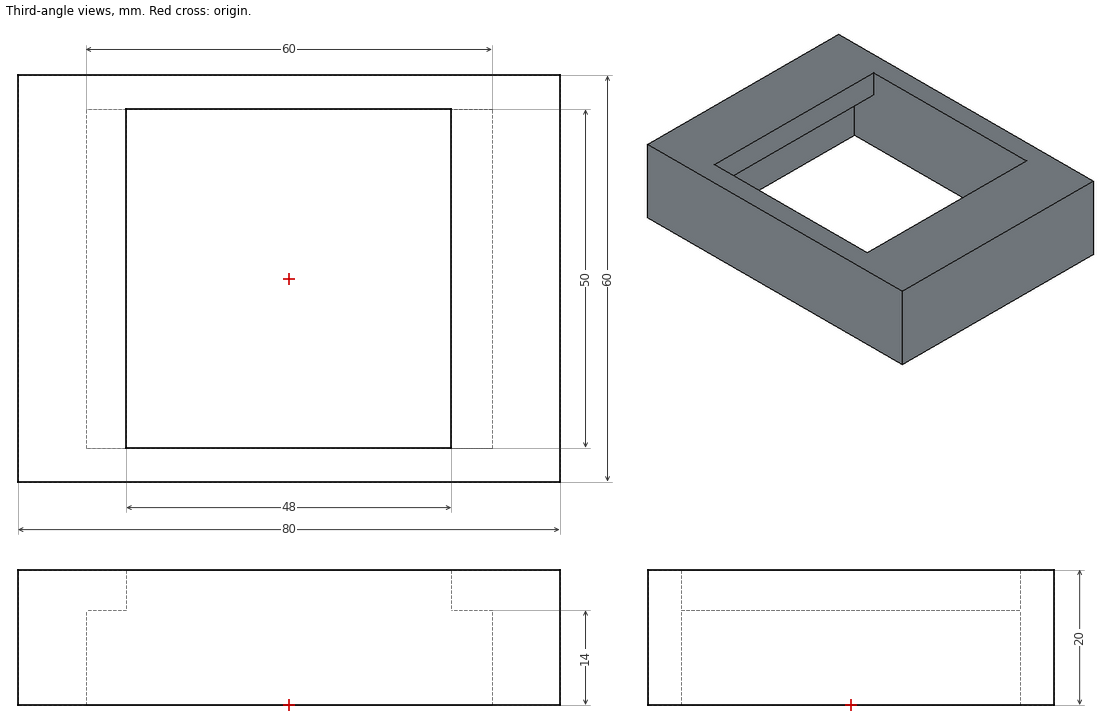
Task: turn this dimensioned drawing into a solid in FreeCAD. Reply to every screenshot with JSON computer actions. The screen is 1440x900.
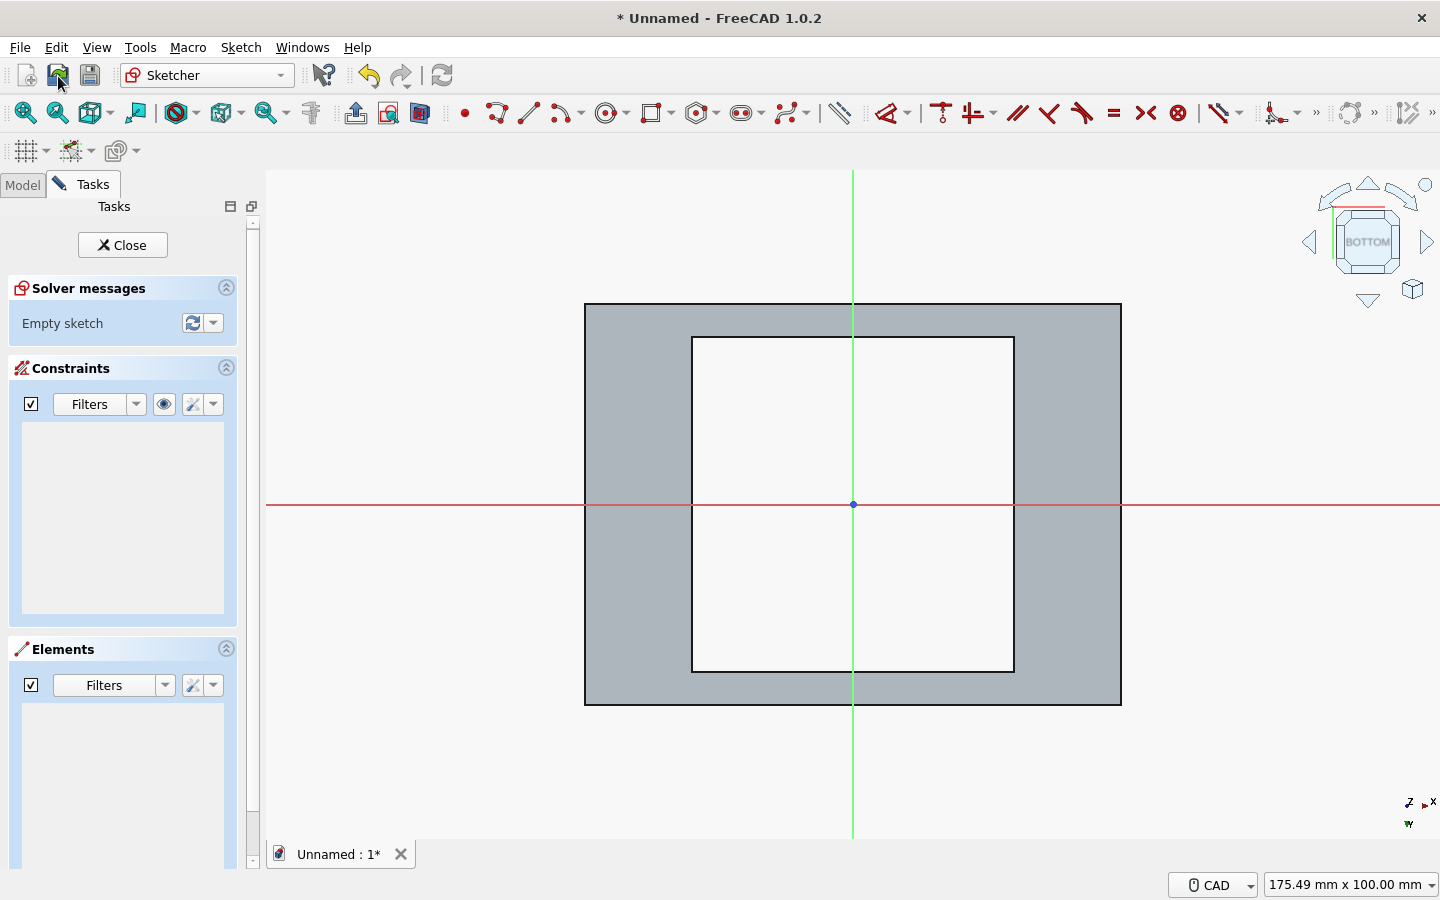
{"action": "key", "text": "g v"}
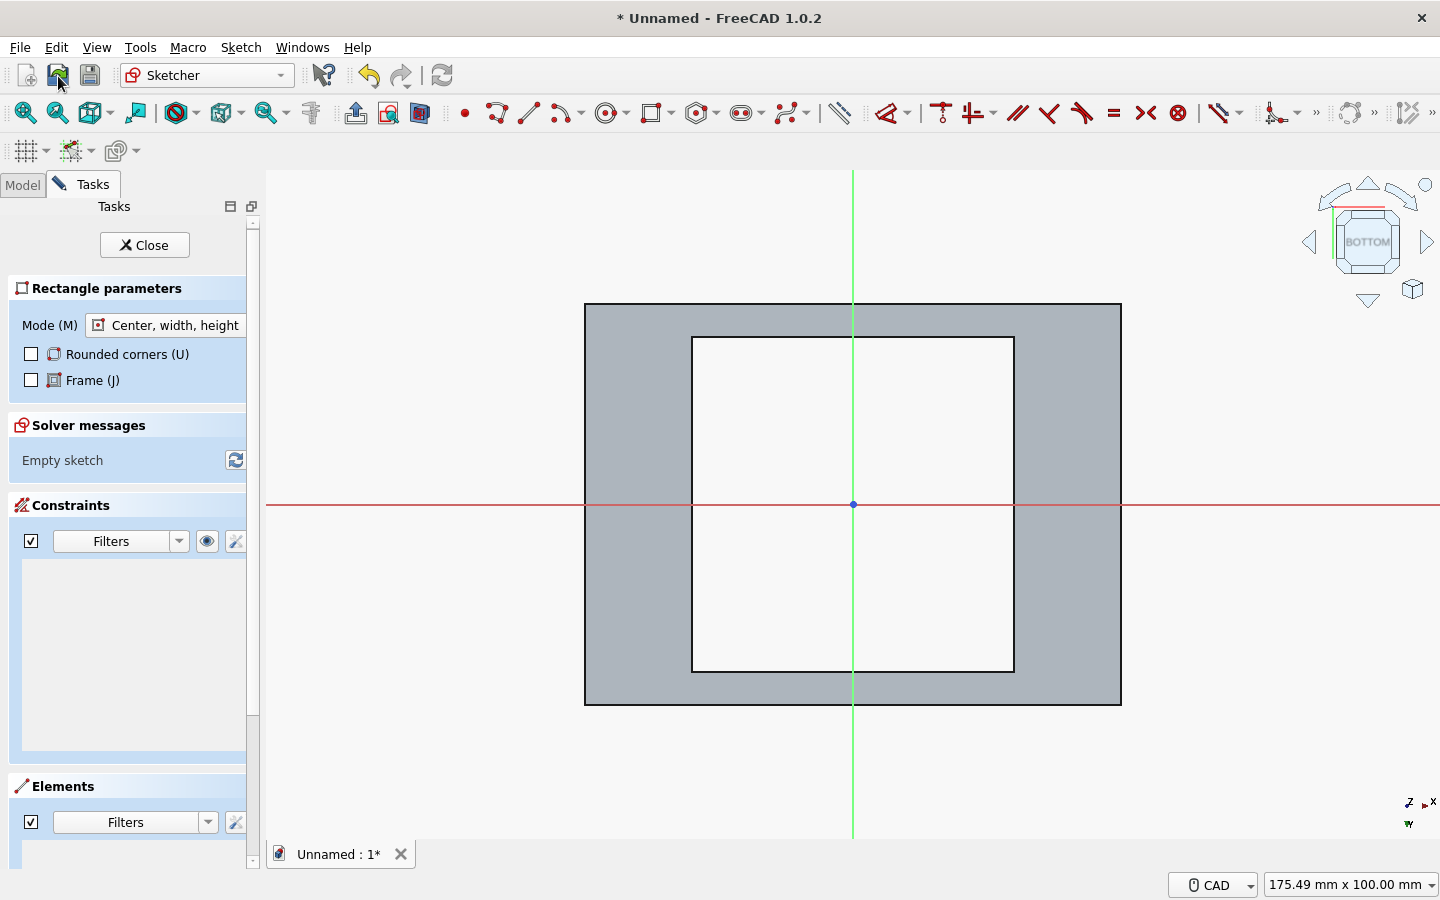
{"action": "left_click", "coordinate": [853, 504]}
{"action": "mouse_move", "coordinate": [1054, 337]}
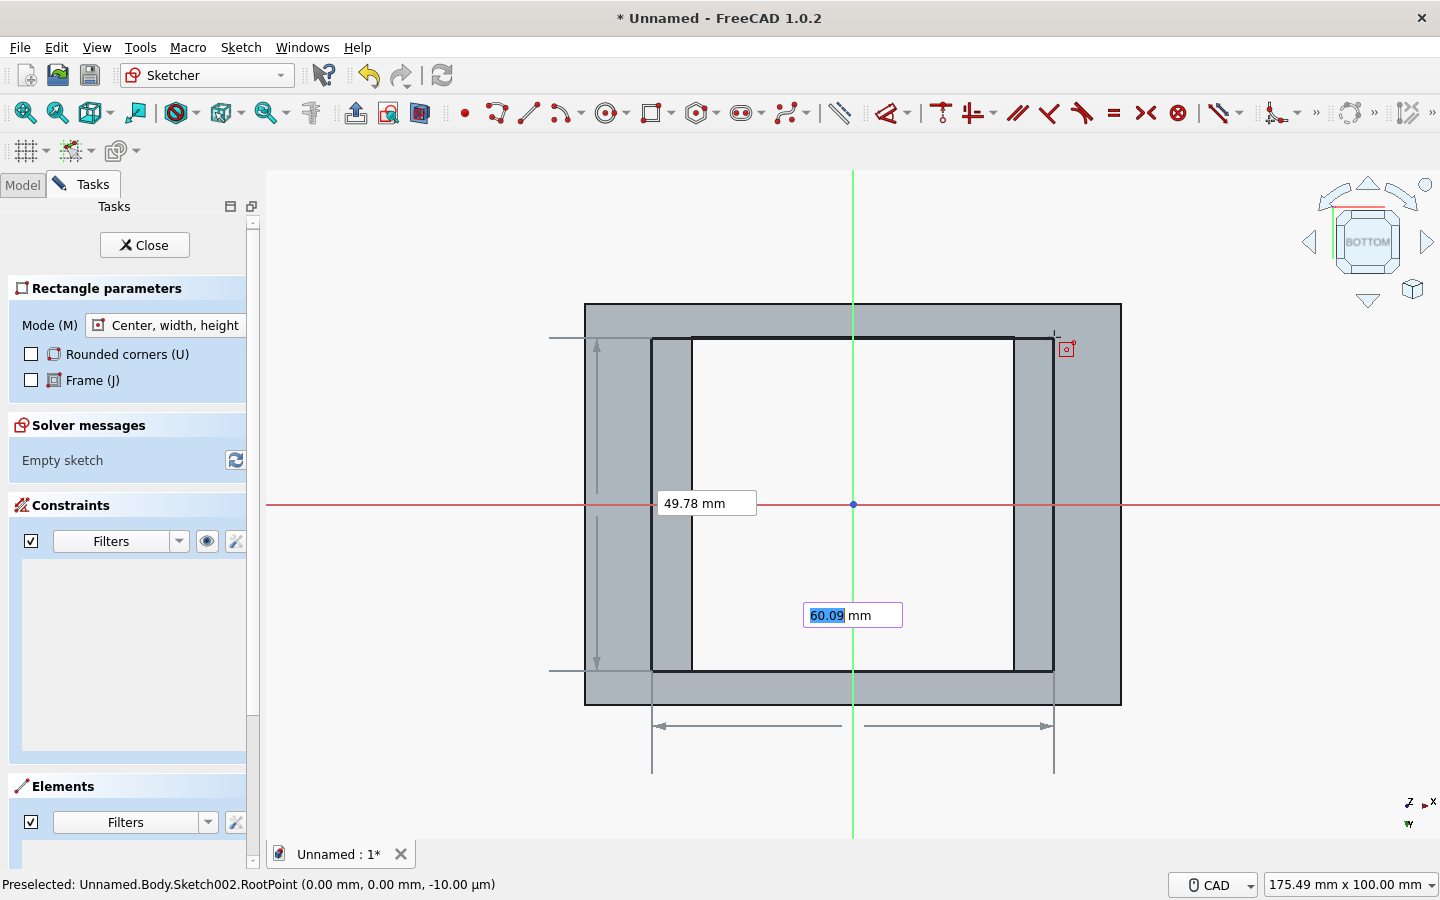
{"action": "type", "text": "60"}
{"action": "key", "text": "Tab"}
{"action": "type", "text": "50"}
{"action": "key", "text": "Return"}
{"action": "key", "text": "Escape"}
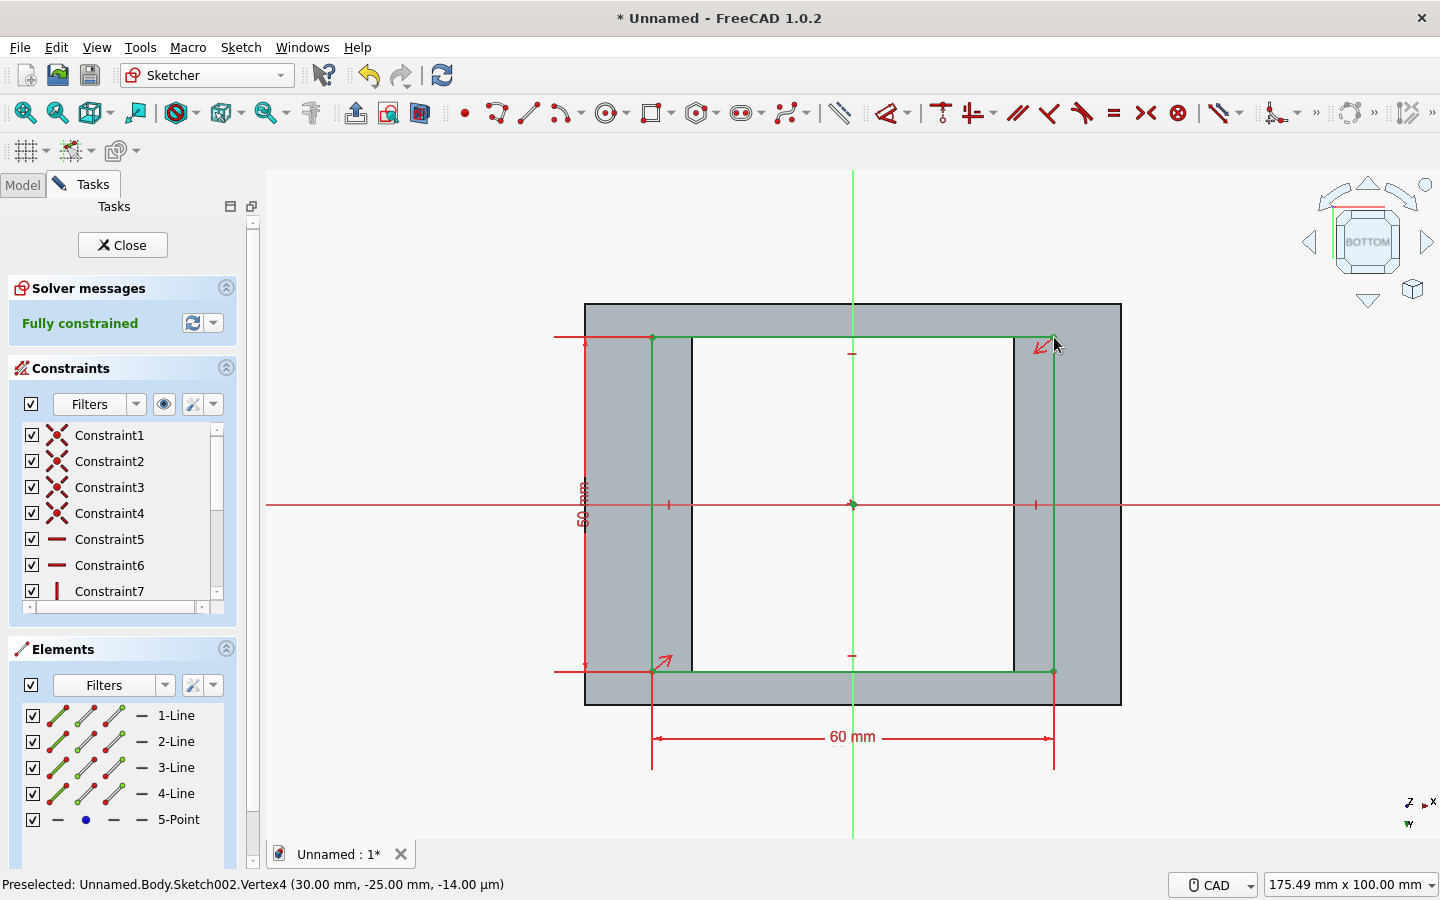
{"action": "left_click", "coordinate": [123, 245]}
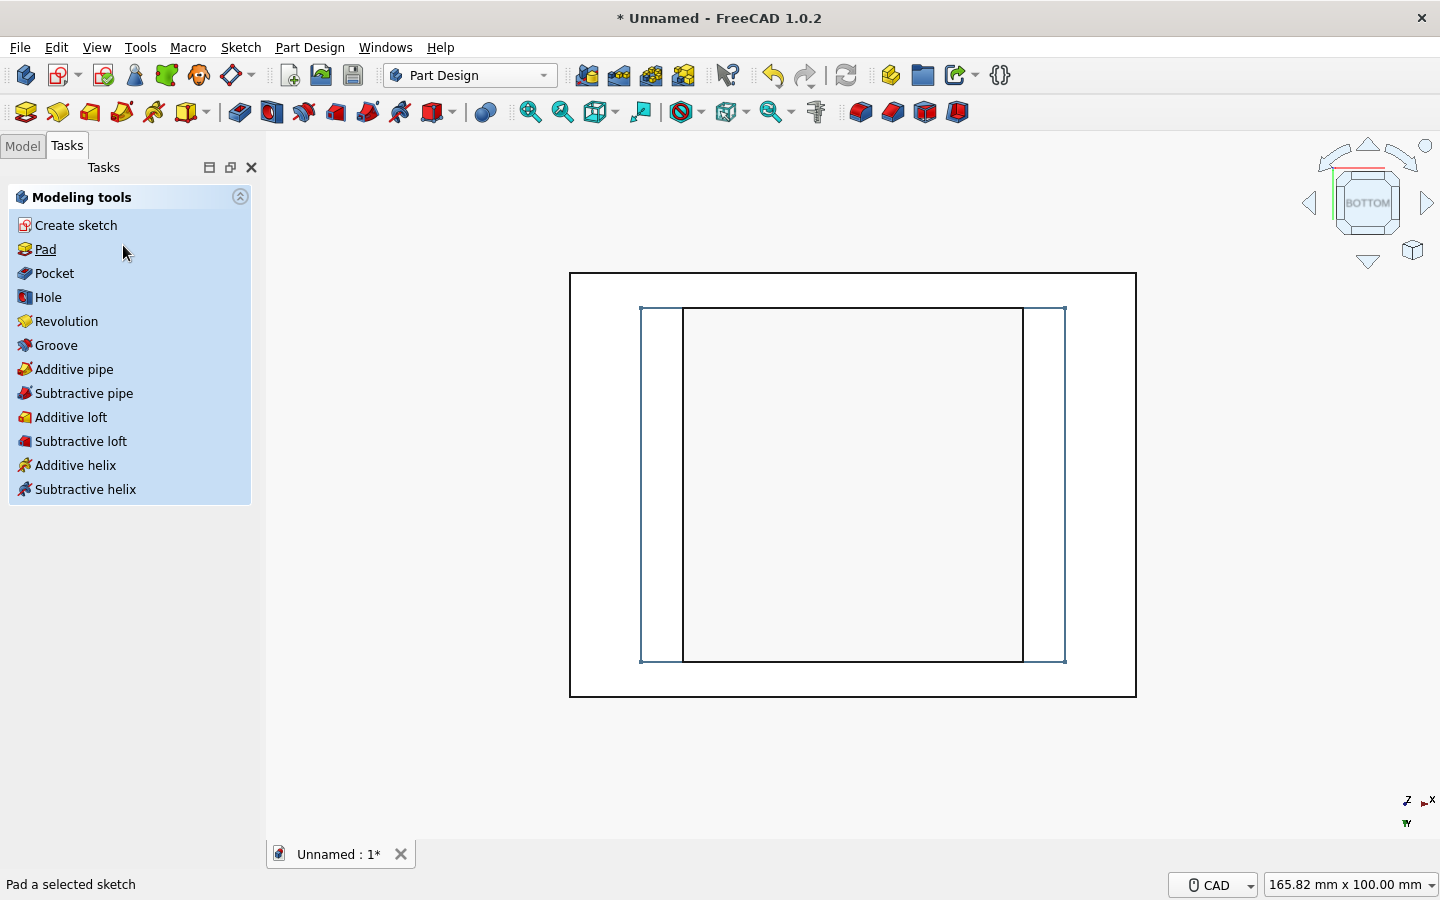
{"action": "left_click", "coordinate": [240, 112]}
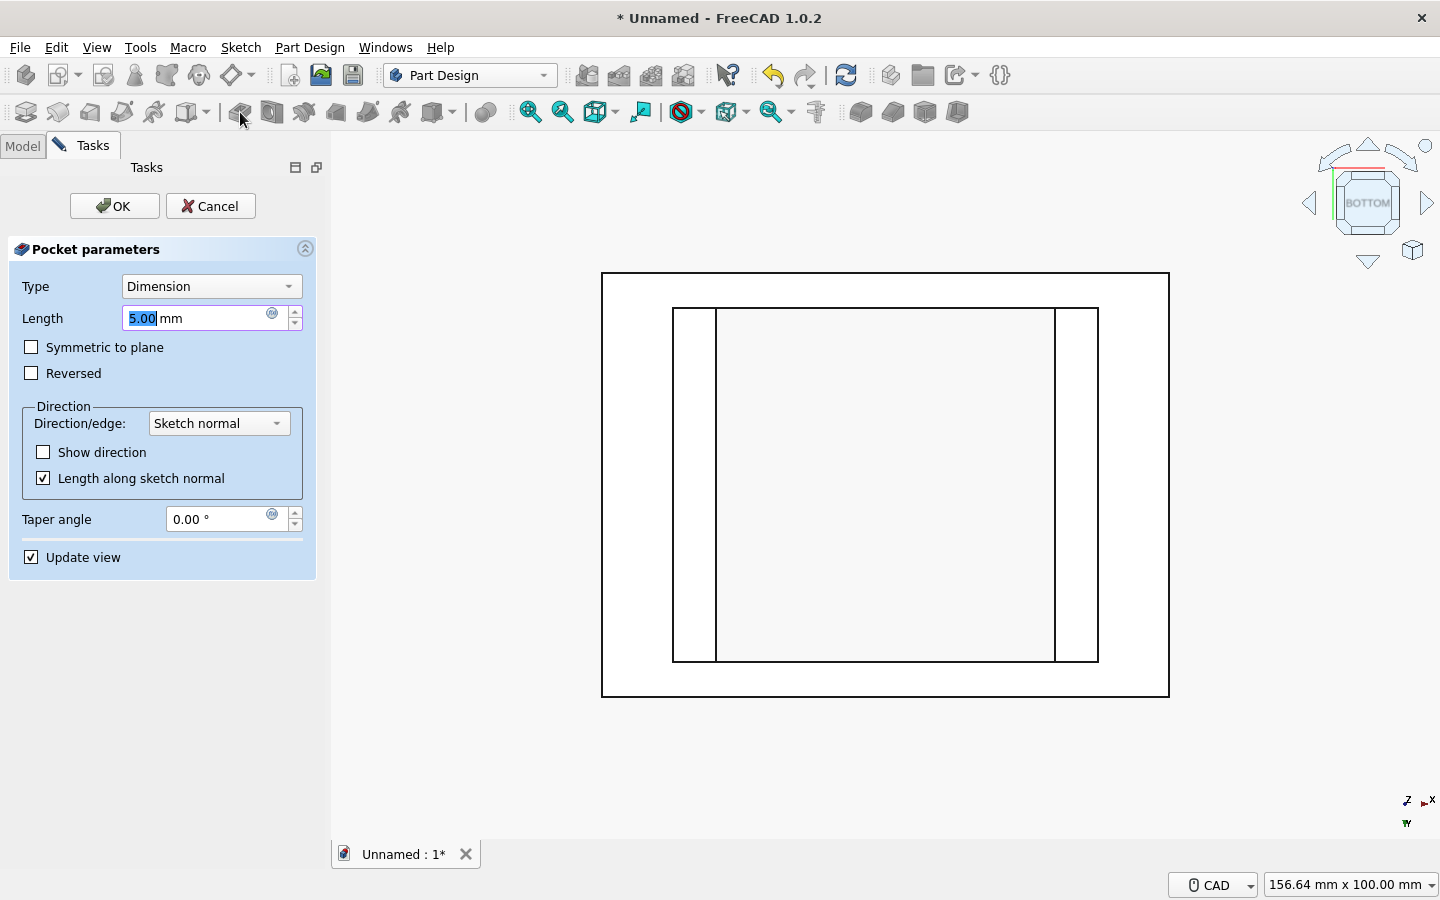
{"action": "type", "text": "14"}
{"action": "key", "text": "Tab"}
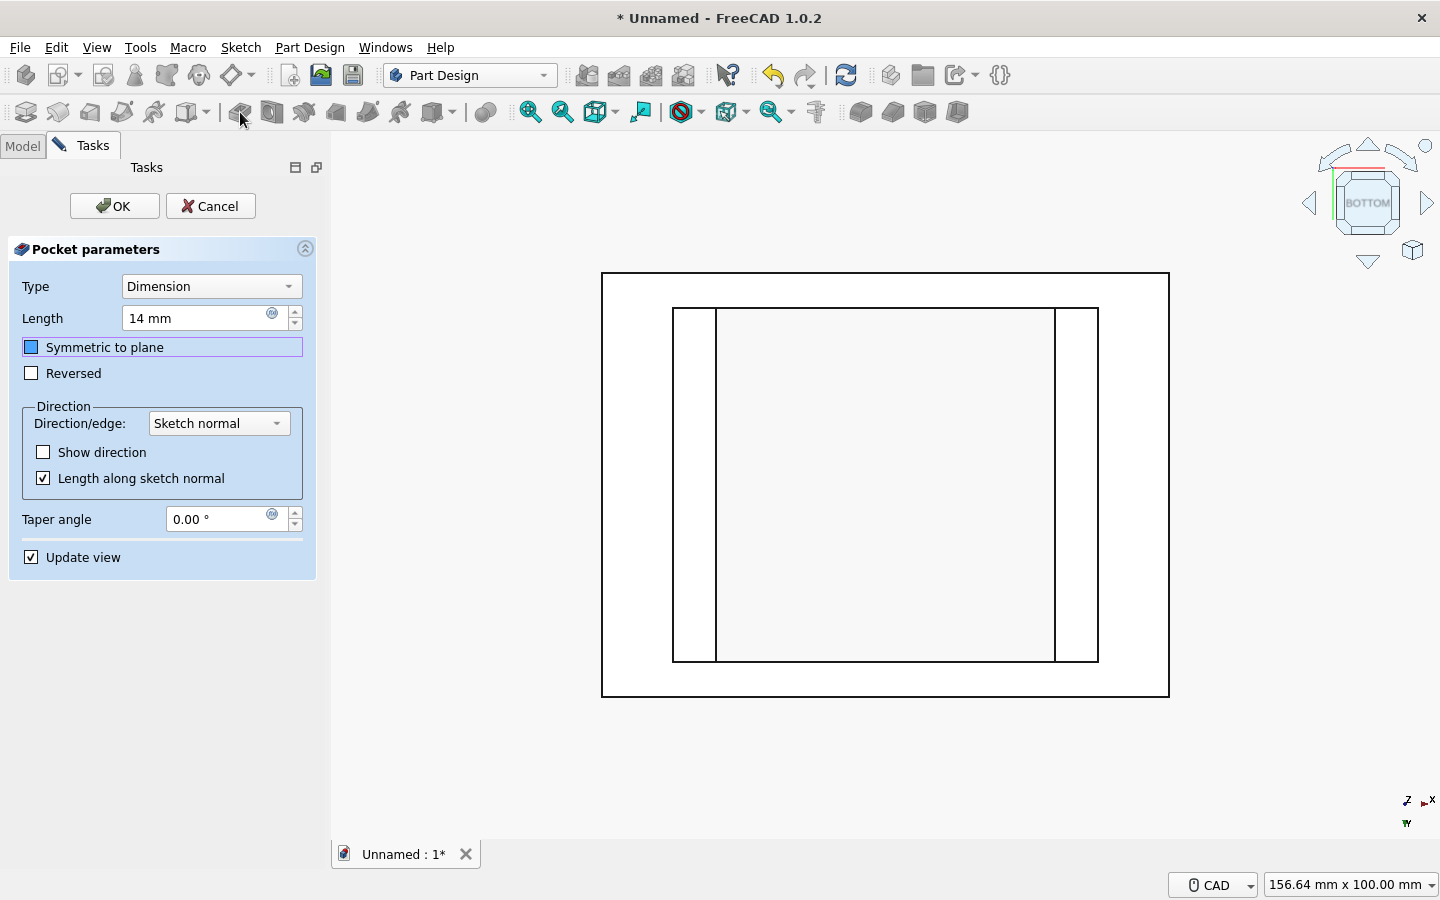
{"action": "left_click", "coordinate": [115, 206]}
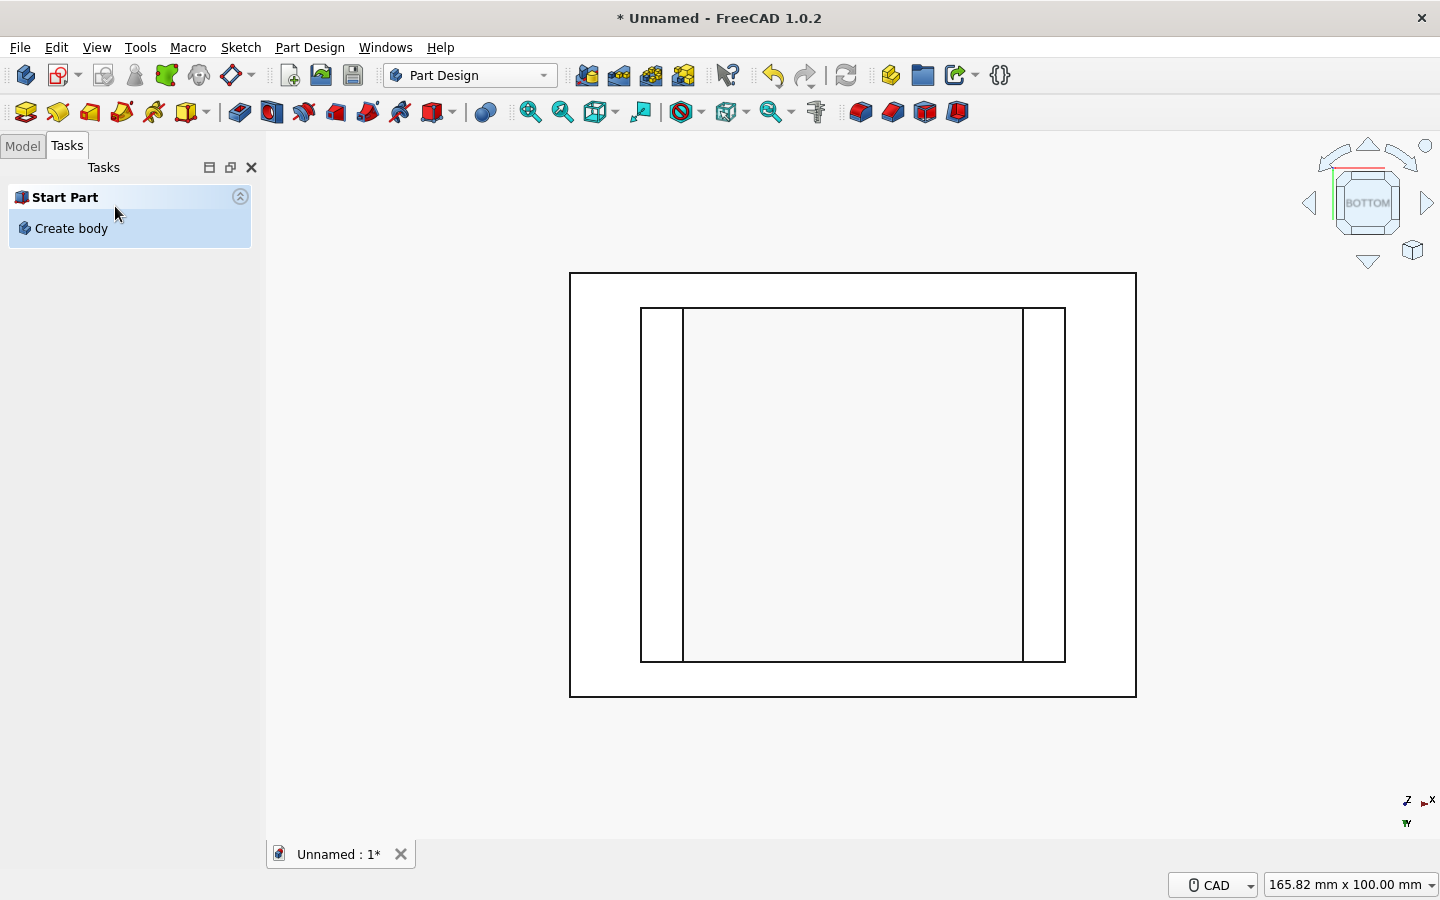
{"action": "key", "text": "0"}